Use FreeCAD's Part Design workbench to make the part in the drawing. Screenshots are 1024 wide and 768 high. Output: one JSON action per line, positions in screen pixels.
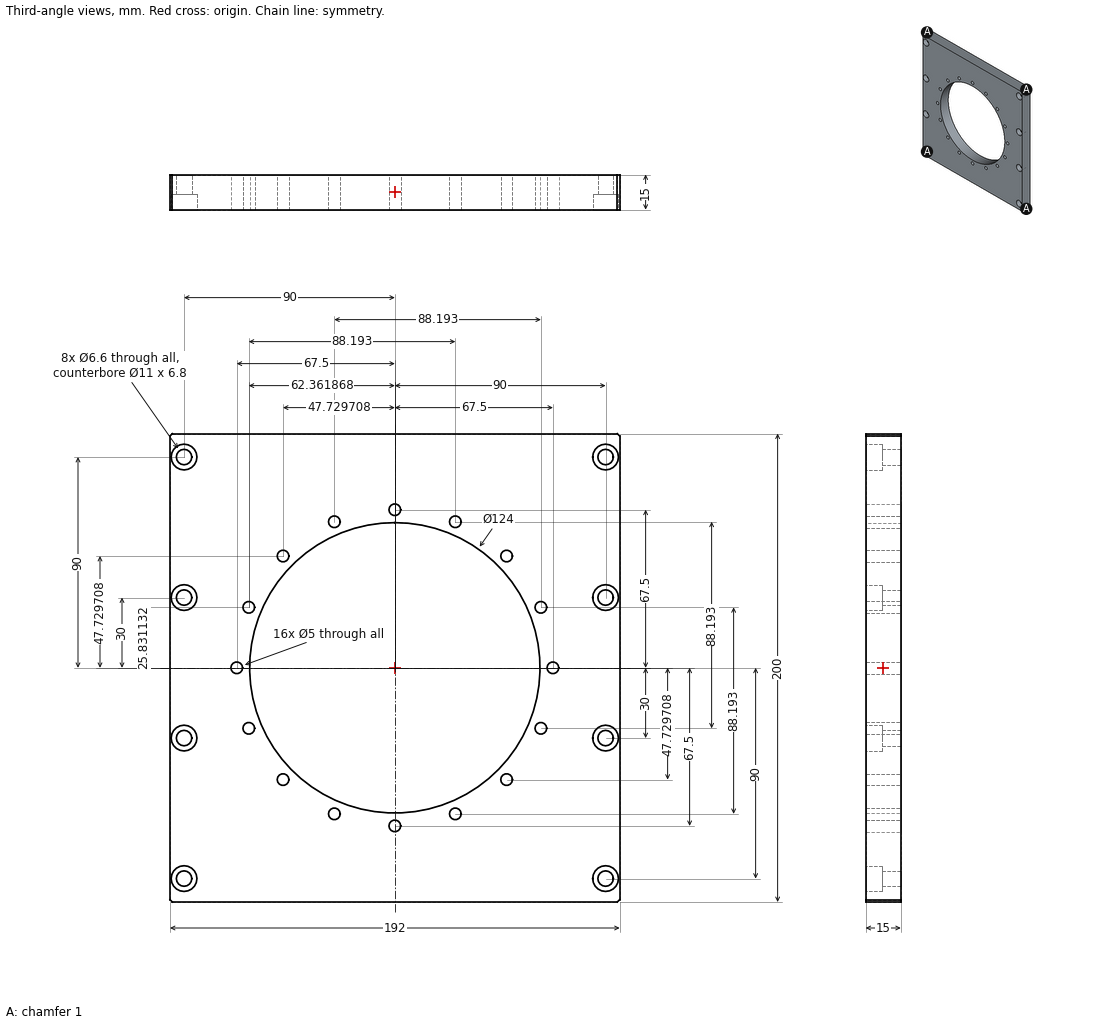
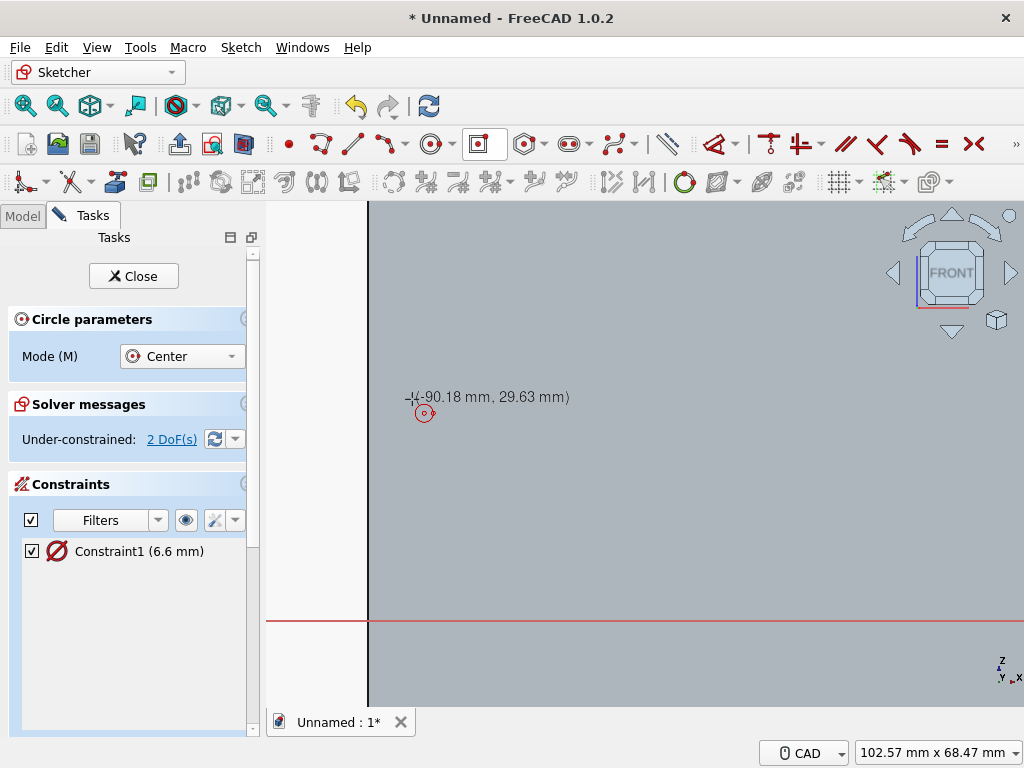
{"action": "scroll", "coordinate": [412, 399], "scroll_direction": "down", "scroll_amount": 7}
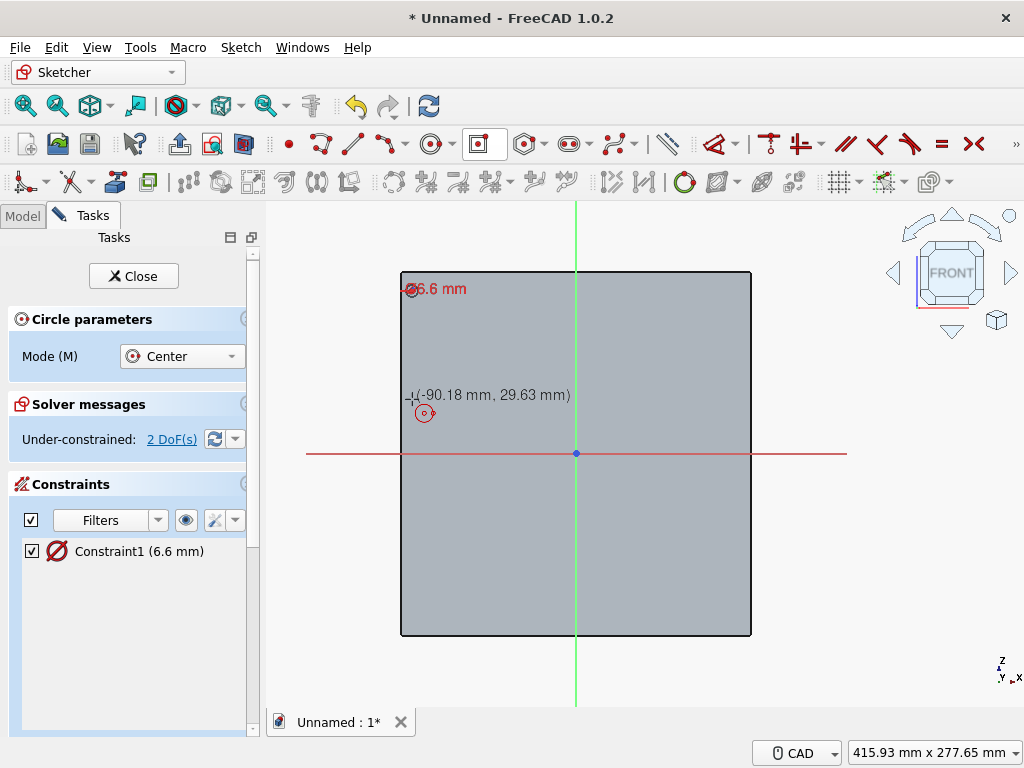
{"action": "left_click", "coordinate": [412, 399]}
{"action": "mouse_move", "coordinate": [417, 395]}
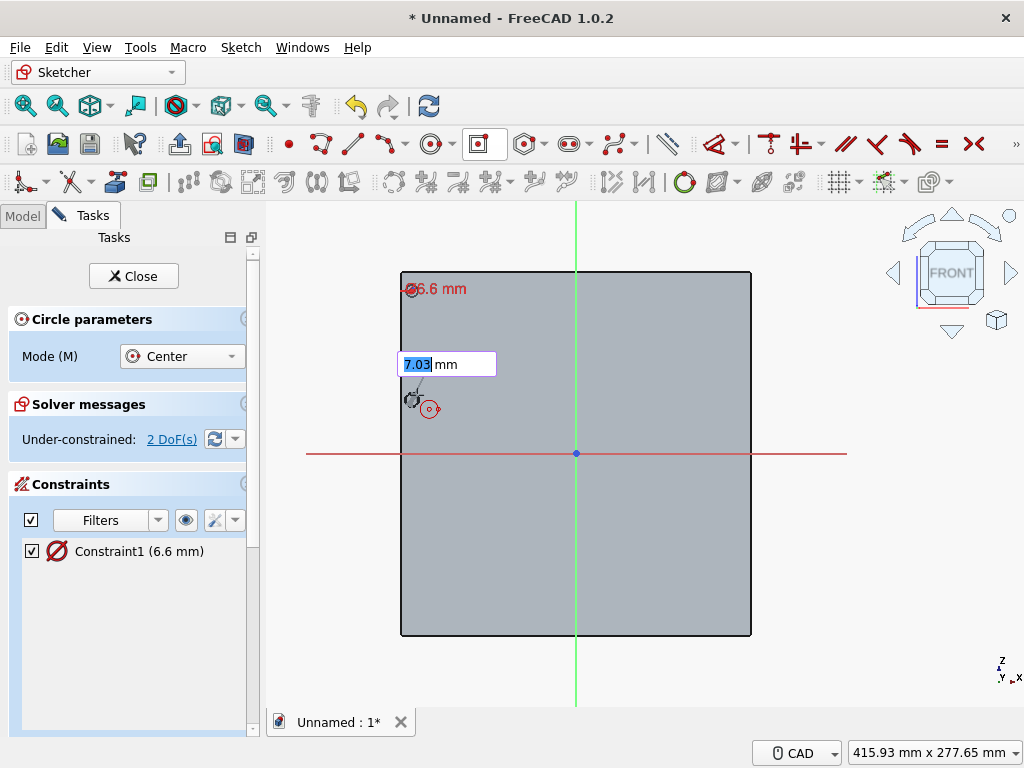
{"action": "type", "text": "6.6"}
{"action": "key", "text": "Return"}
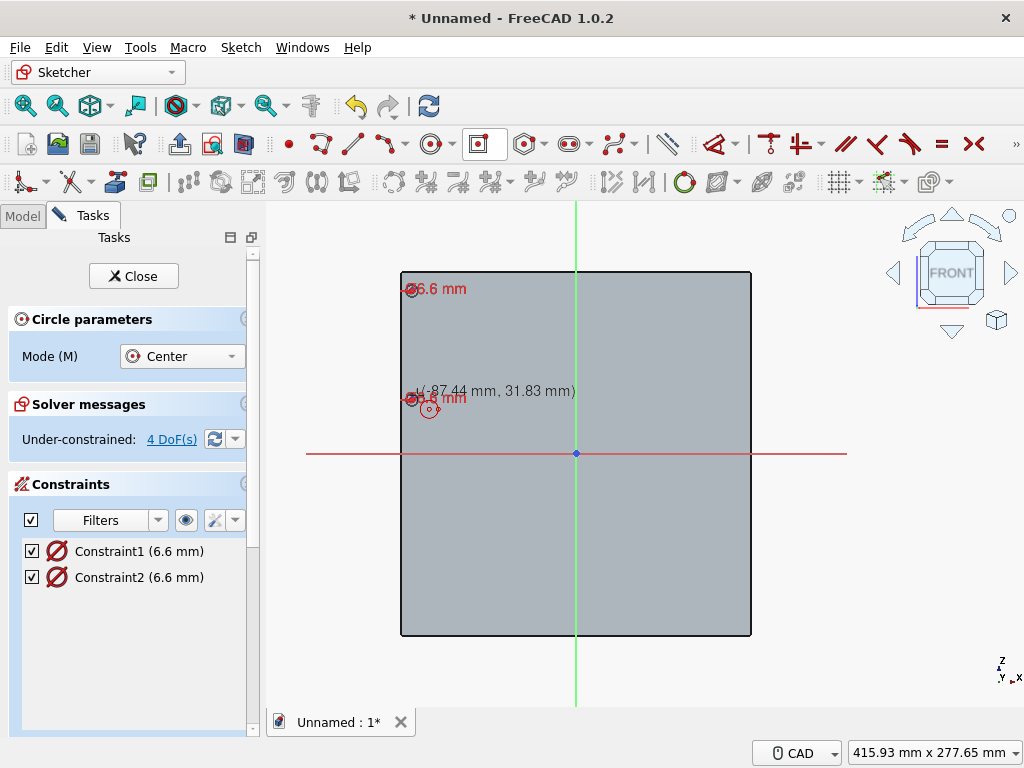
{"action": "scroll", "coordinate": [740, 399], "scroll_direction": "up", "scroll_amount": 7}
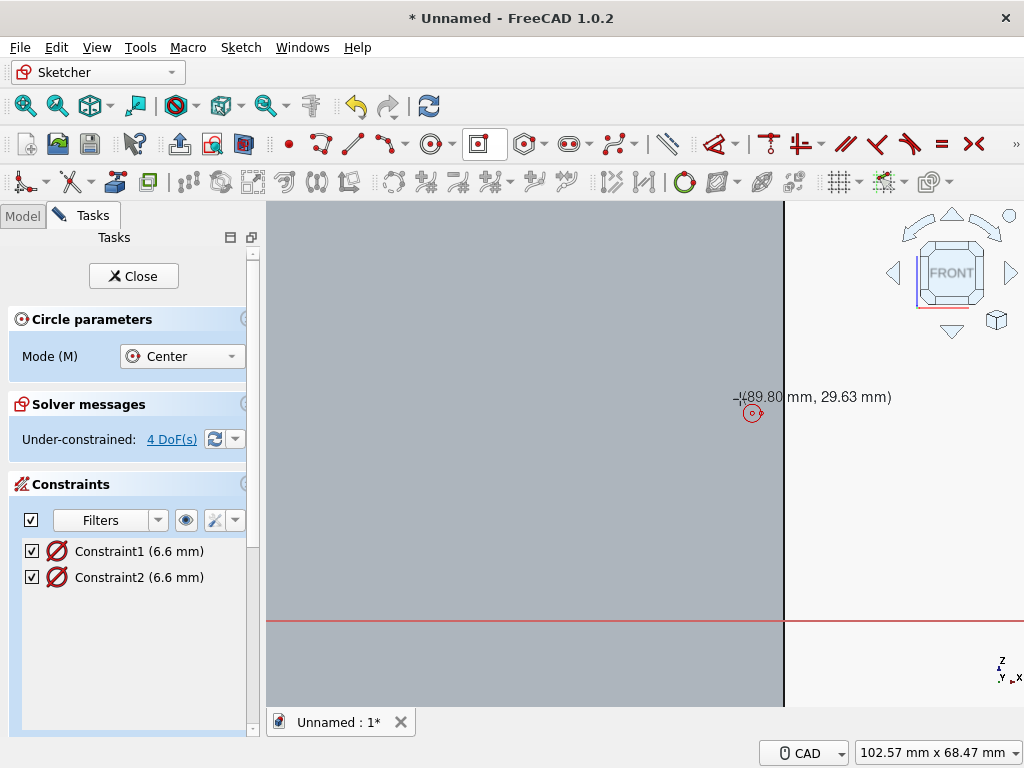
{"action": "scroll", "coordinate": [741, 399], "scroll_direction": "down", "scroll_amount": 7}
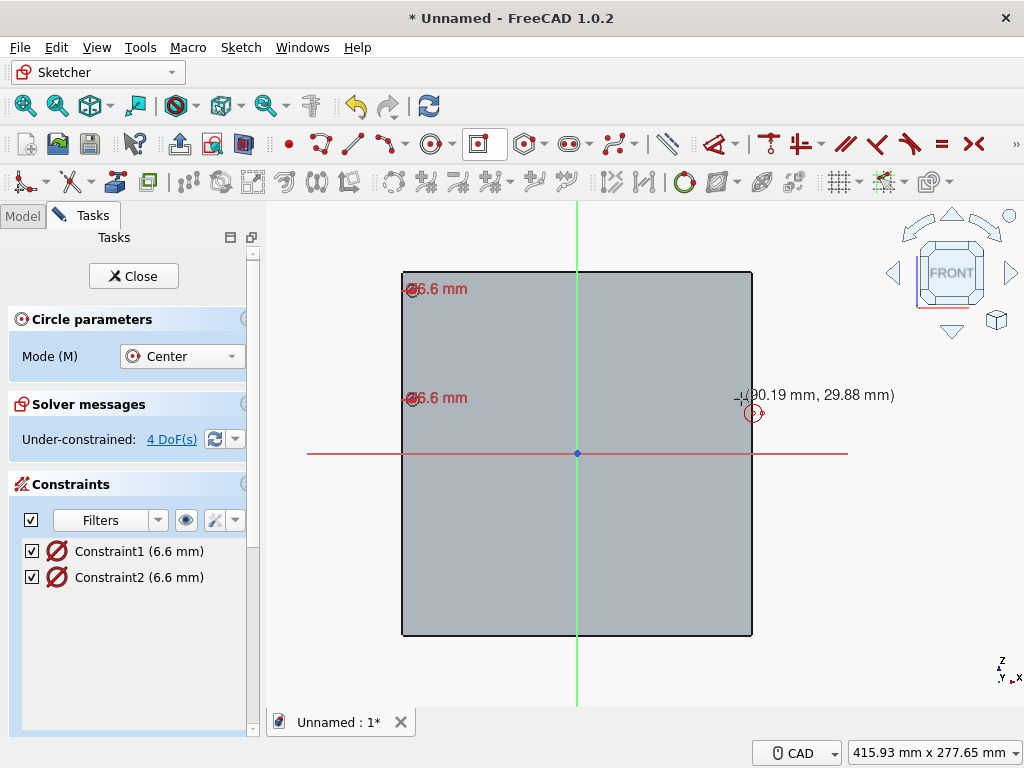
{"action": "left_click", "coordinate": [741, 399]}
{"action": "mouse_move", "coordinate": [745, 395]}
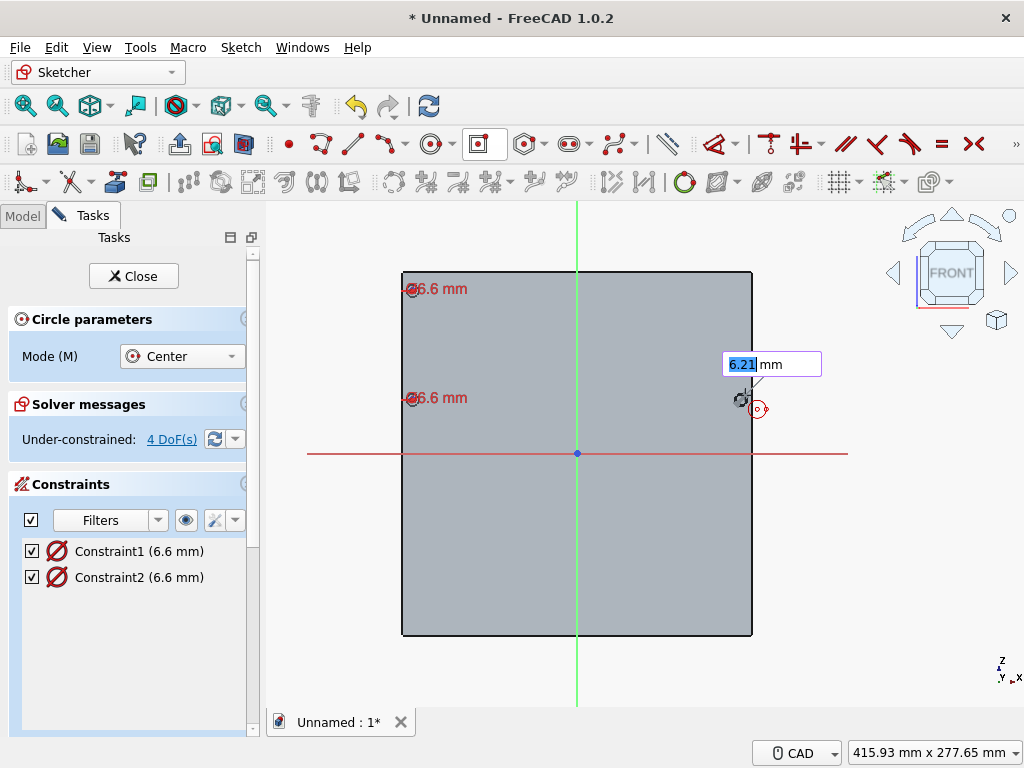
{"action": "type", "text": "6.6"}
{"action": "key", "text": "Return"}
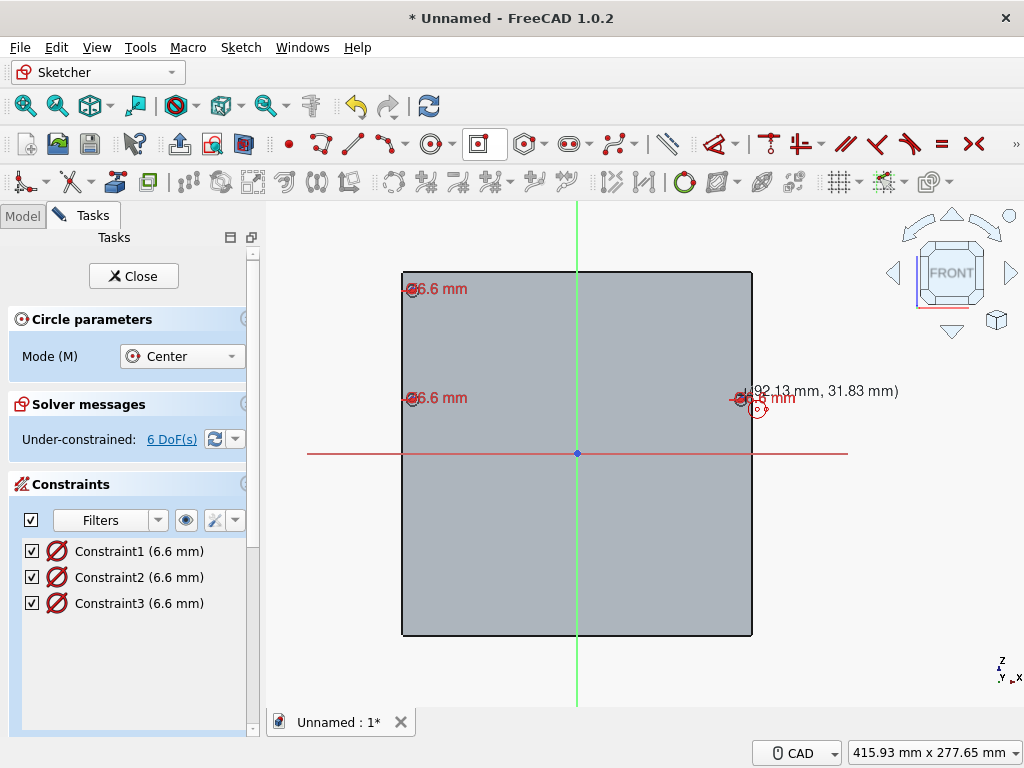
{"action": "scroll", "coordinate": [741, 290], "scroll_direction": "up", "scroll_amount": 7}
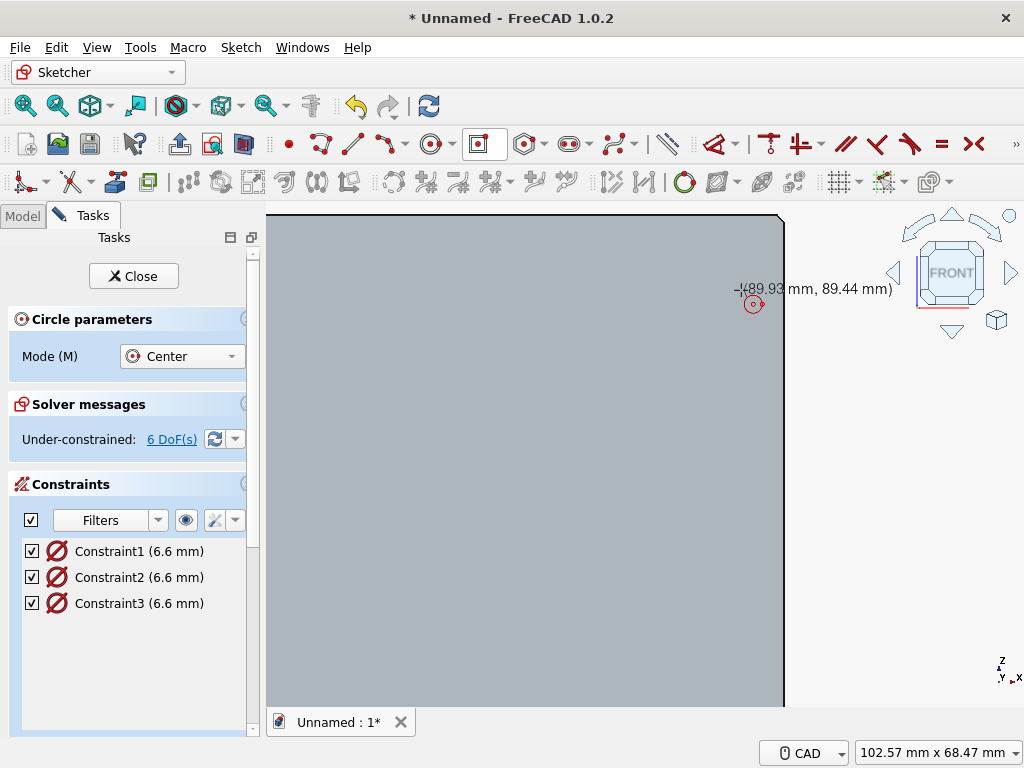
{"action": "scroll", "coordinate": [741, 290], "scroll_direction": "down", "scroll_amount": 7}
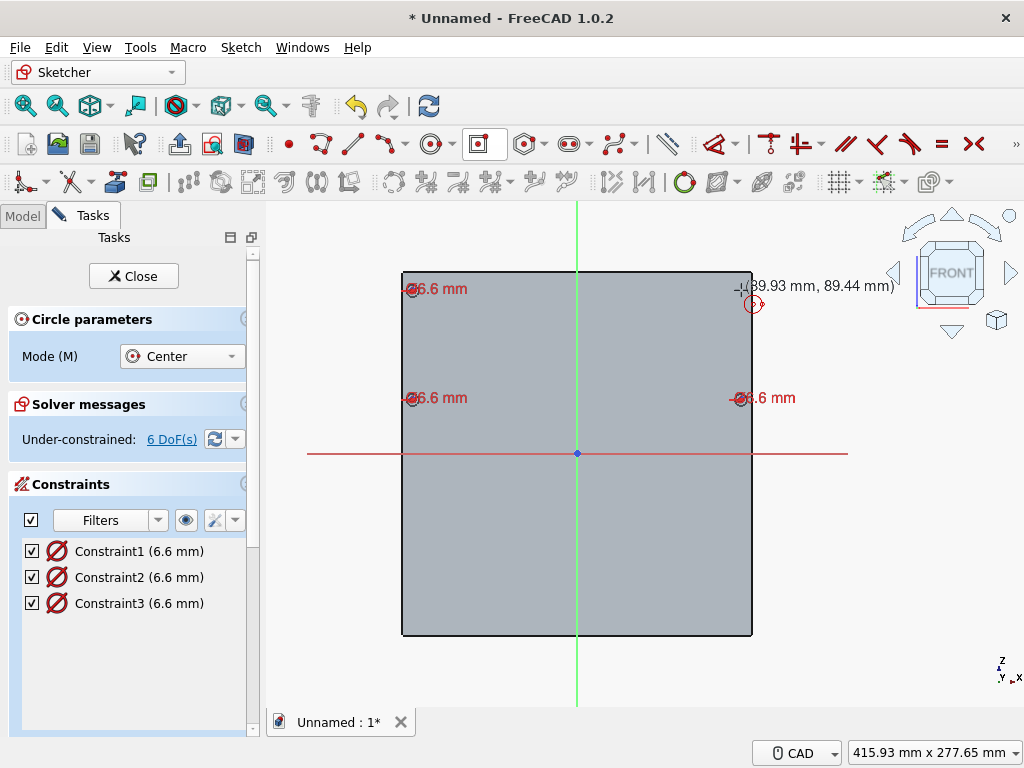
{"action": "left_click", "coordinate": [741, 290]}
{"action": "mouse_move", "coordinate": [745, 286]}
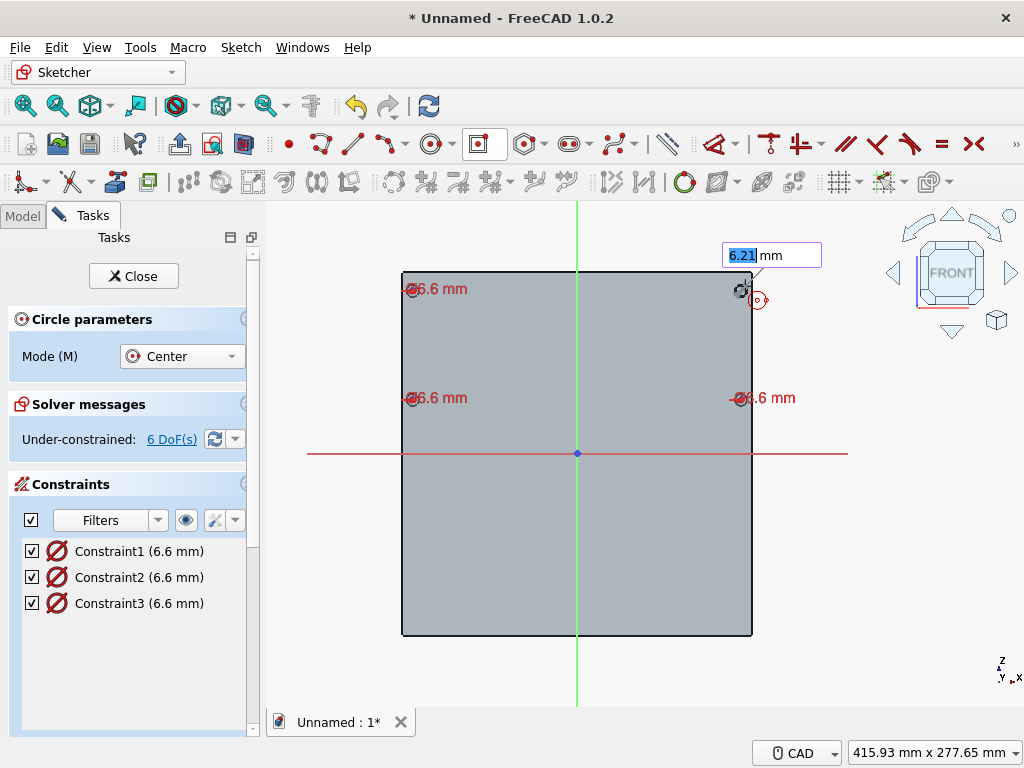
{"action": "type", "text": "6.6"}
{"action": "key", "text": "Return"}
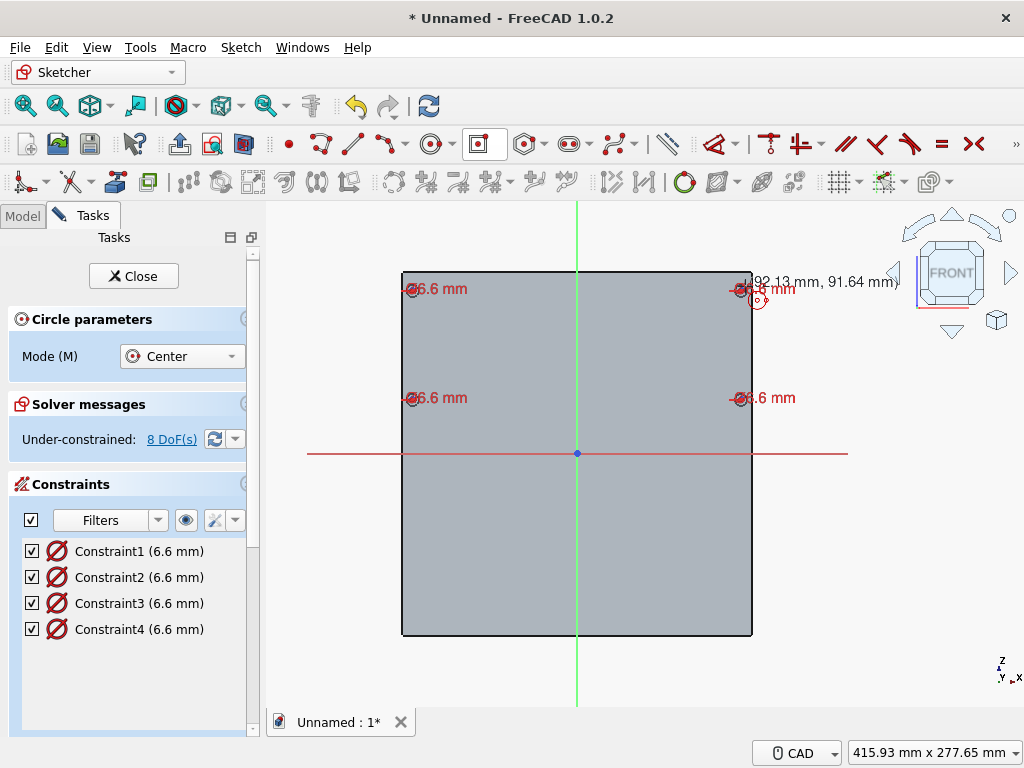
{"action": "scroll", "coordinate": [741, 618], "scroll_direction": "up", "scroll_amount": 7}